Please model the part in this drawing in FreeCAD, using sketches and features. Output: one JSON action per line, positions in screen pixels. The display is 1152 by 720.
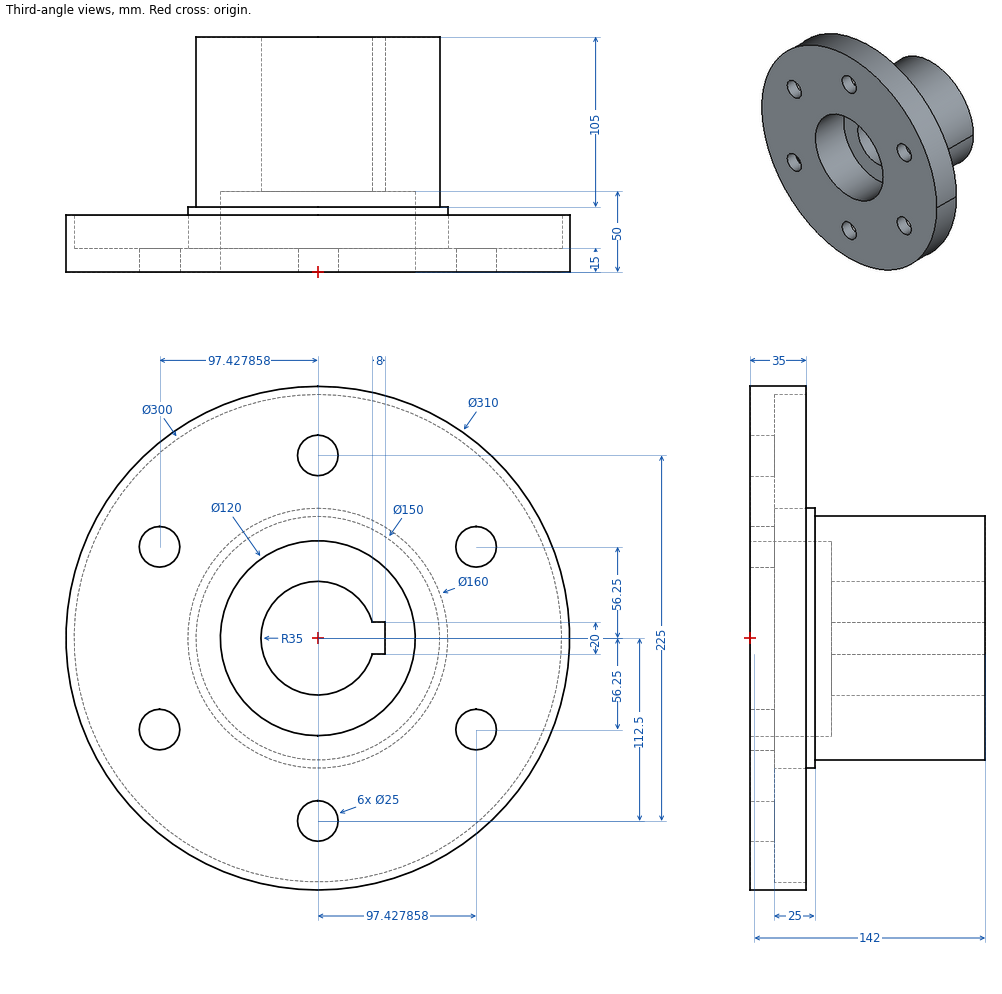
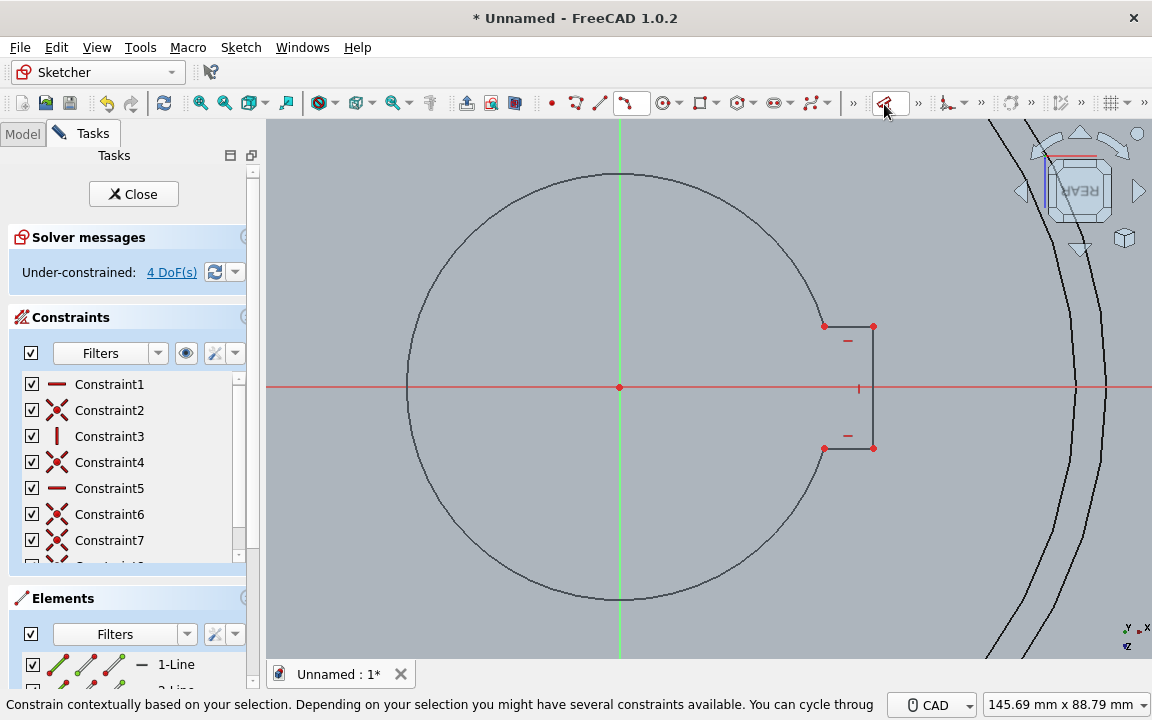
{"action": "left_click", "coordinate": [532, 193]}
{"action": "left_click", "coordinate": [519, 164]}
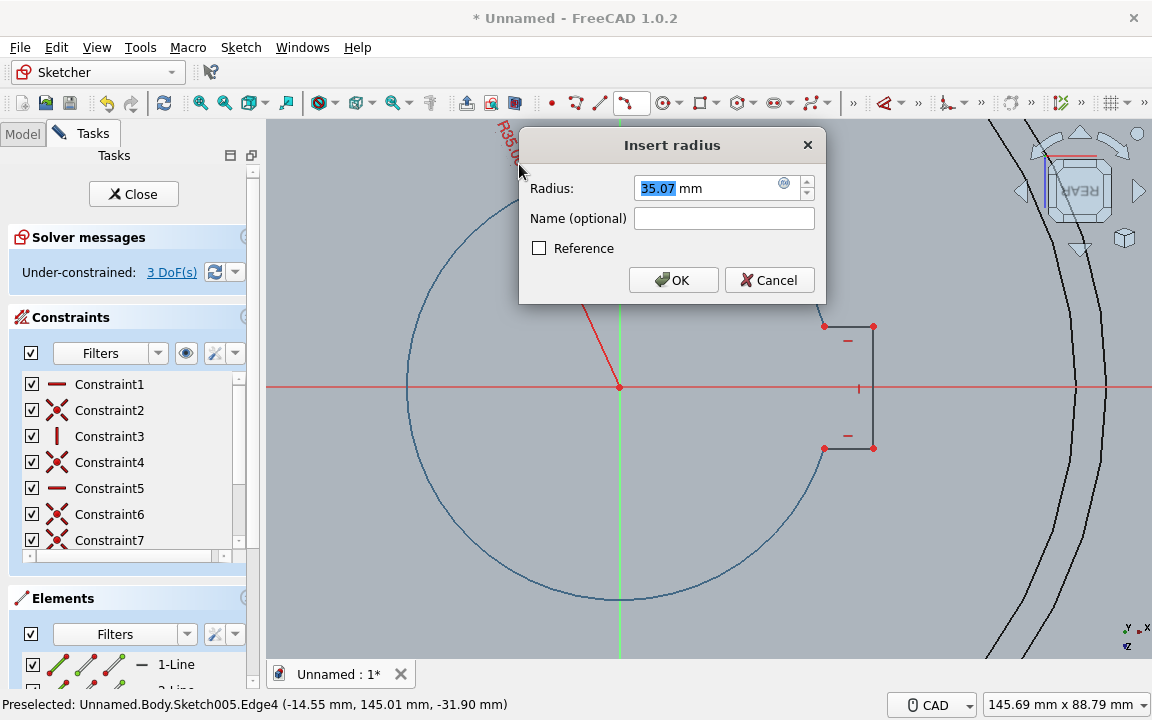
{"action": "type", "text": "35"}
{"action": "key", "text": "Return"}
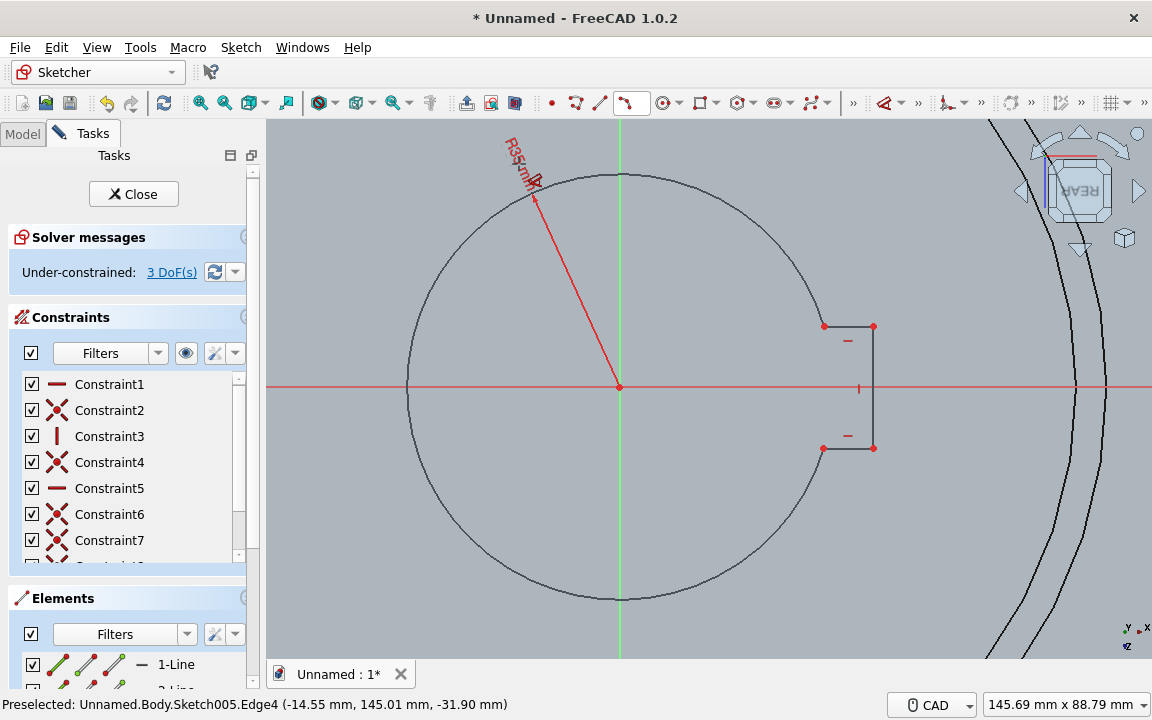
{"action": "left_click", "coordinate": [838, 449]}
{"action": "left_click", "coordinate": [848, 483]}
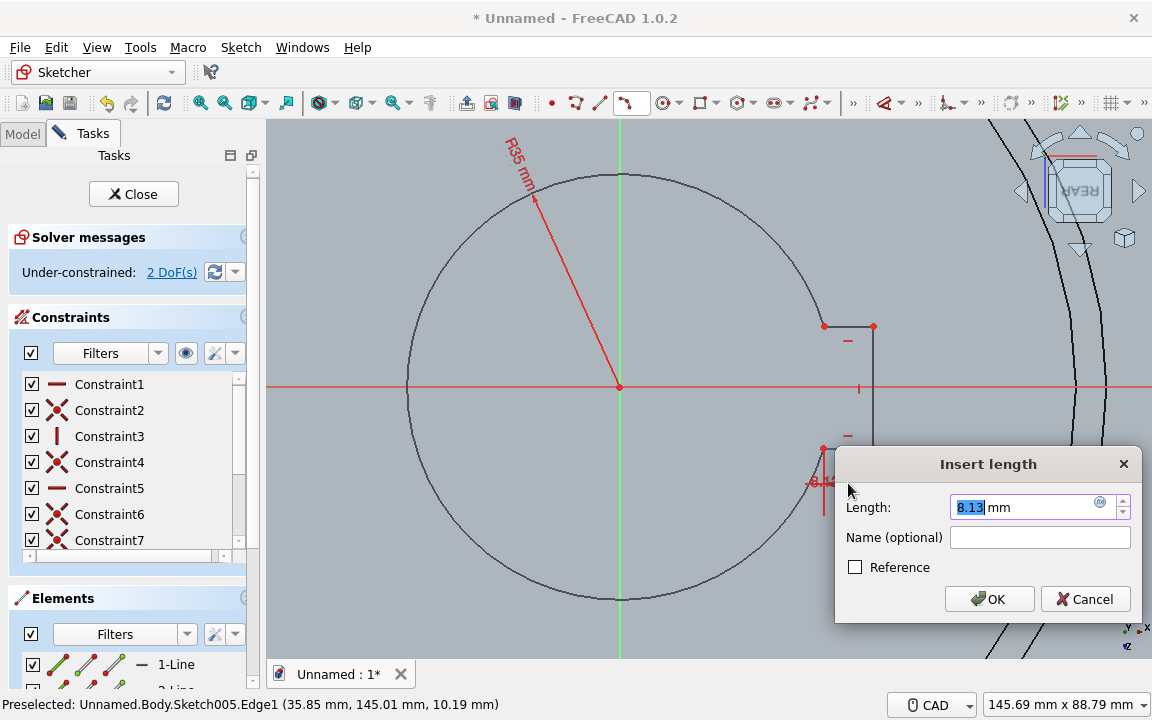
{"action": "type", "text": "8"}
{"action": "key", "text": "Return"}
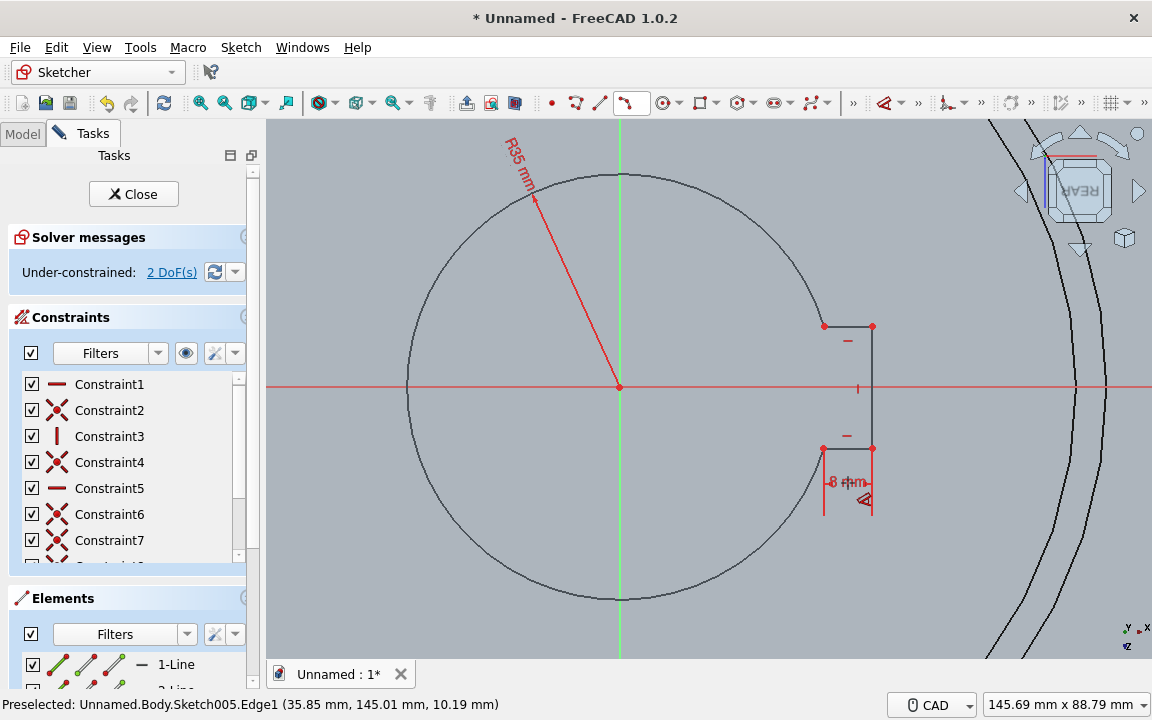
{"action": "left_click", "coordinate": [858, 327]}
{"action": "left_click", "coordinate": [848, 293]}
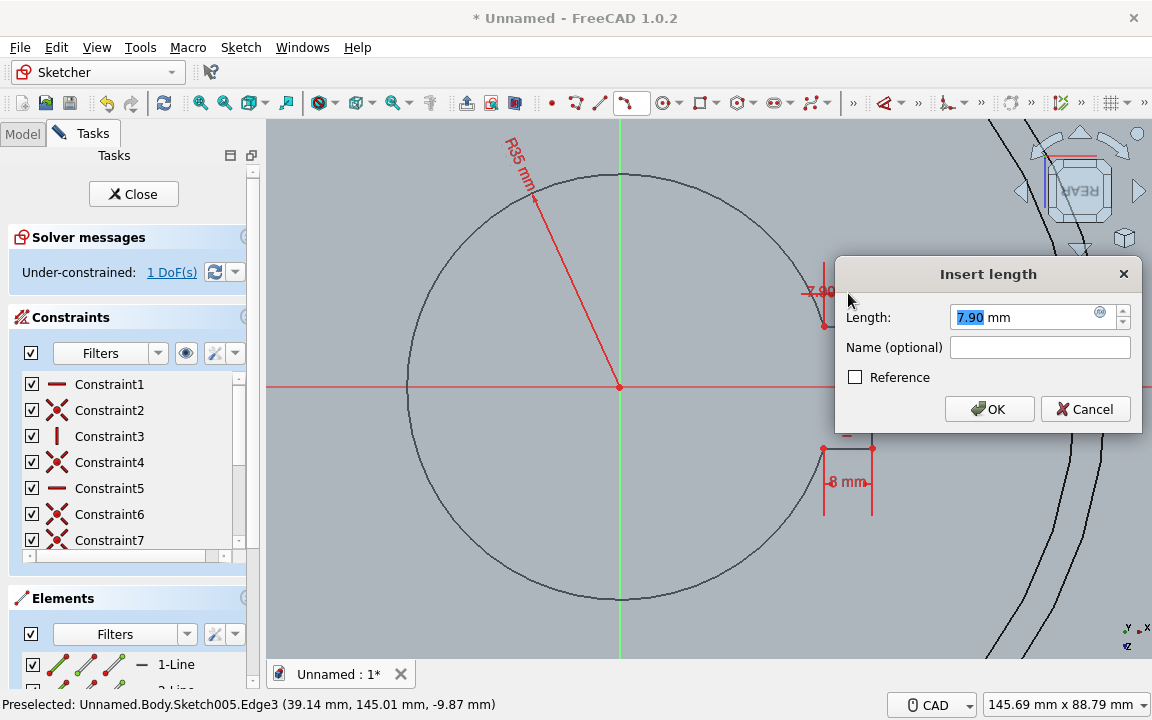
{"action": "type", "text": "8"}
{"action": "key", "text": "Return"}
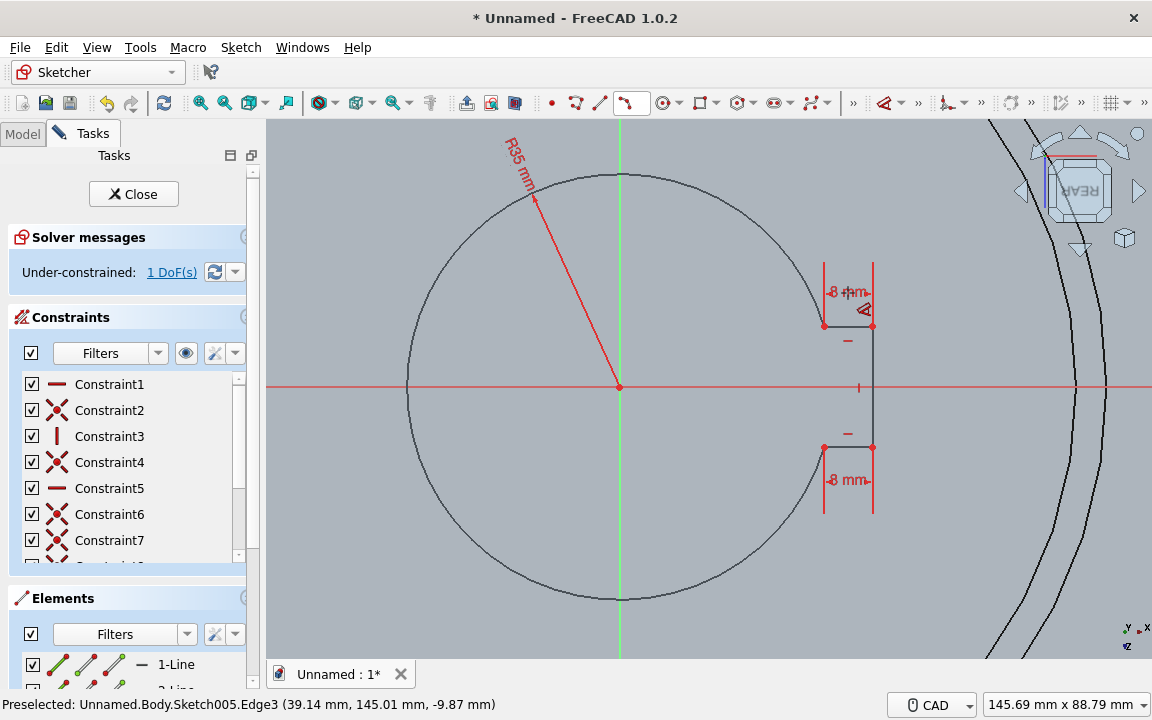
{"action": "left_click", "coordinate": [873, 411]}
{"action": "left_click", "coordinate": [907, 359]}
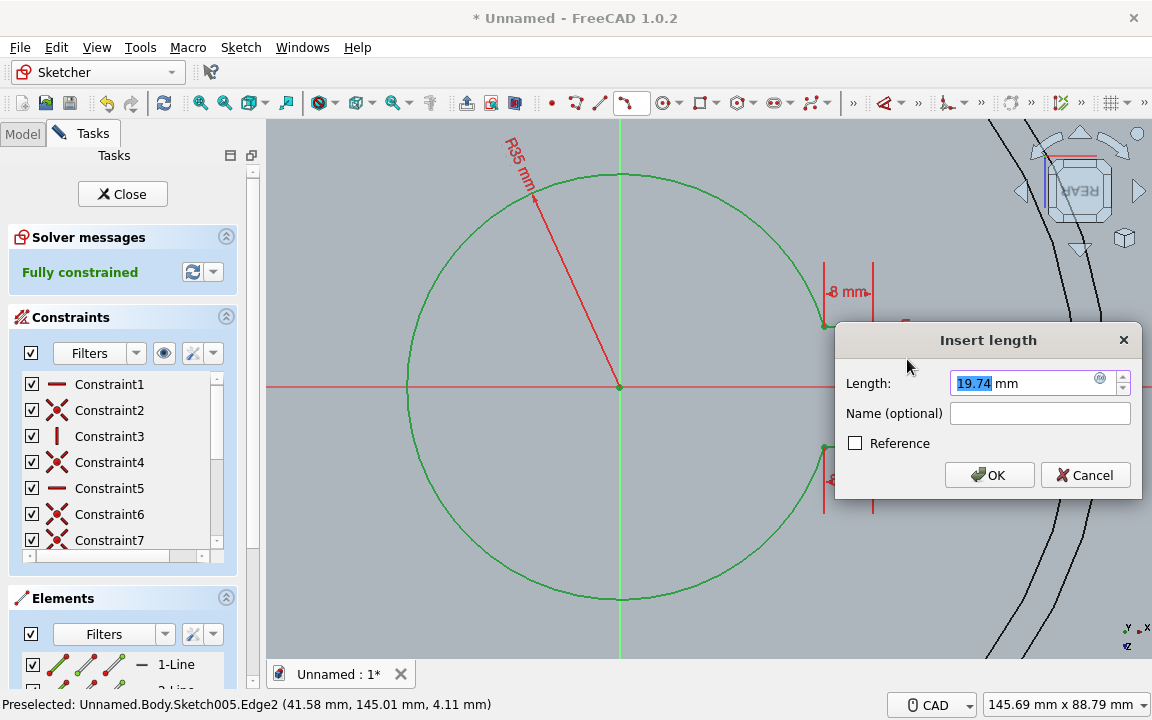
{"action": "type", "text": "20"}
{"action": "key", "text": "Return"}
{"action": "key", "text": "Escape"}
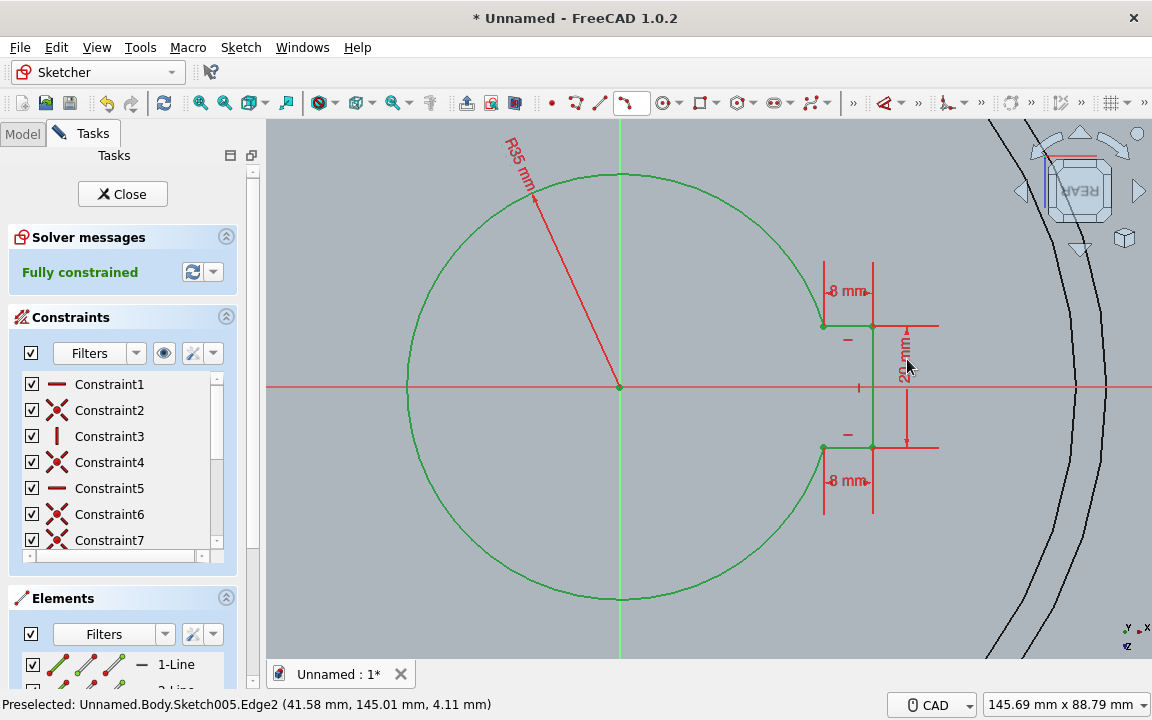
{"action": "left_click", "coordinate": [123, 194]}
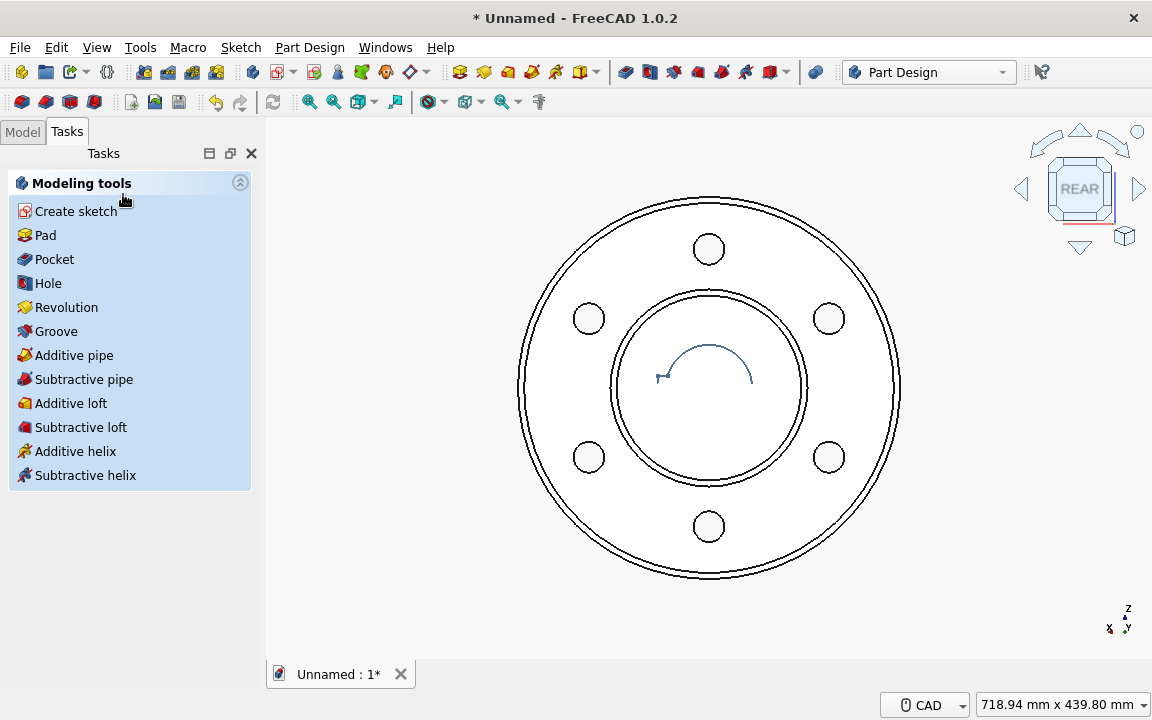
{"action": "left_click", "coordinate": [626, 72]}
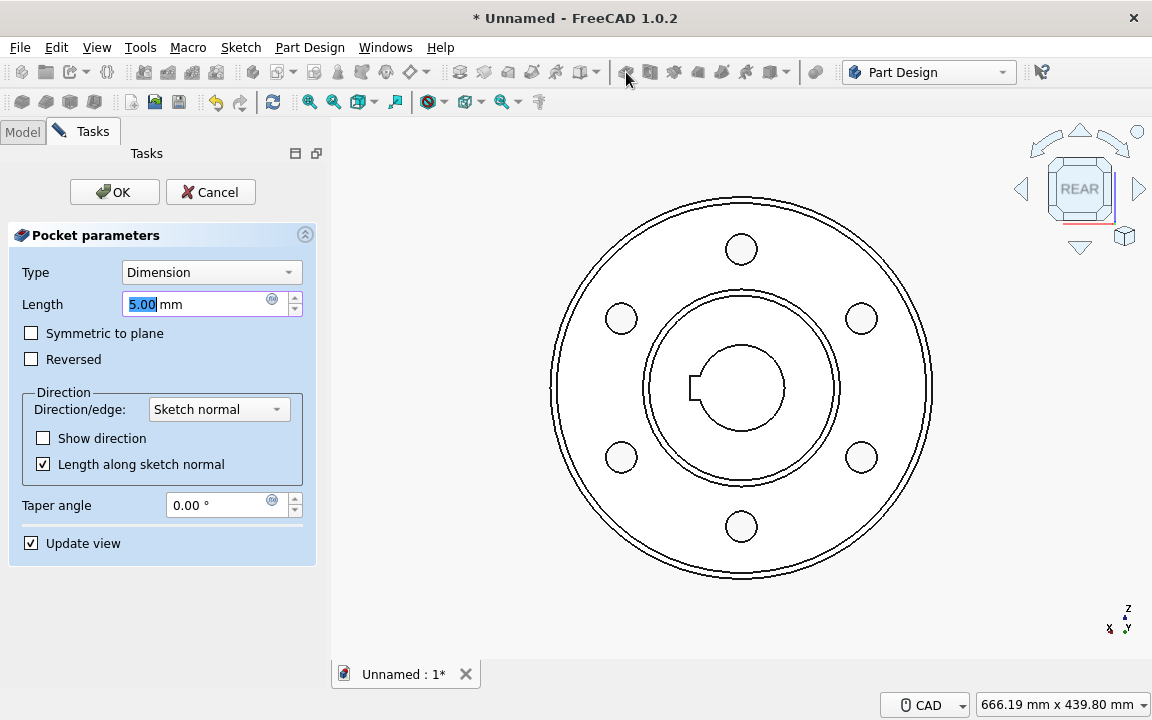
{"action": "type", "text": "142"}
{"action": "key", "text": "Tab"}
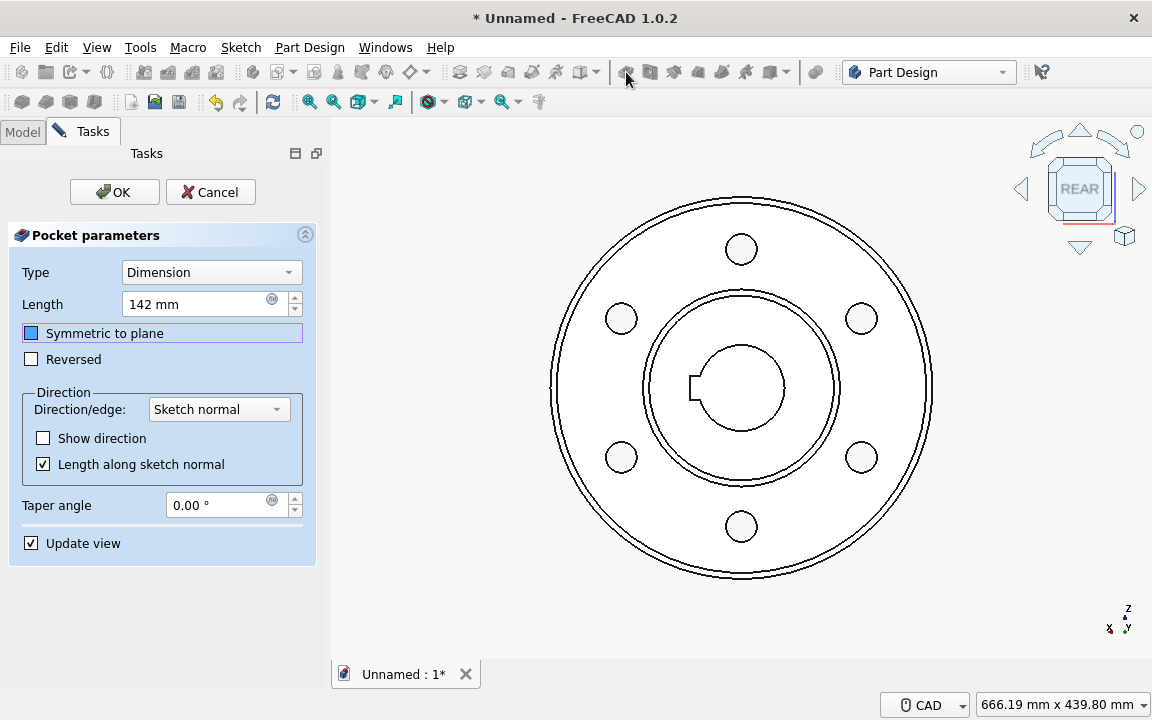
{"action": "left_click", "coordinate": [115, 192]}